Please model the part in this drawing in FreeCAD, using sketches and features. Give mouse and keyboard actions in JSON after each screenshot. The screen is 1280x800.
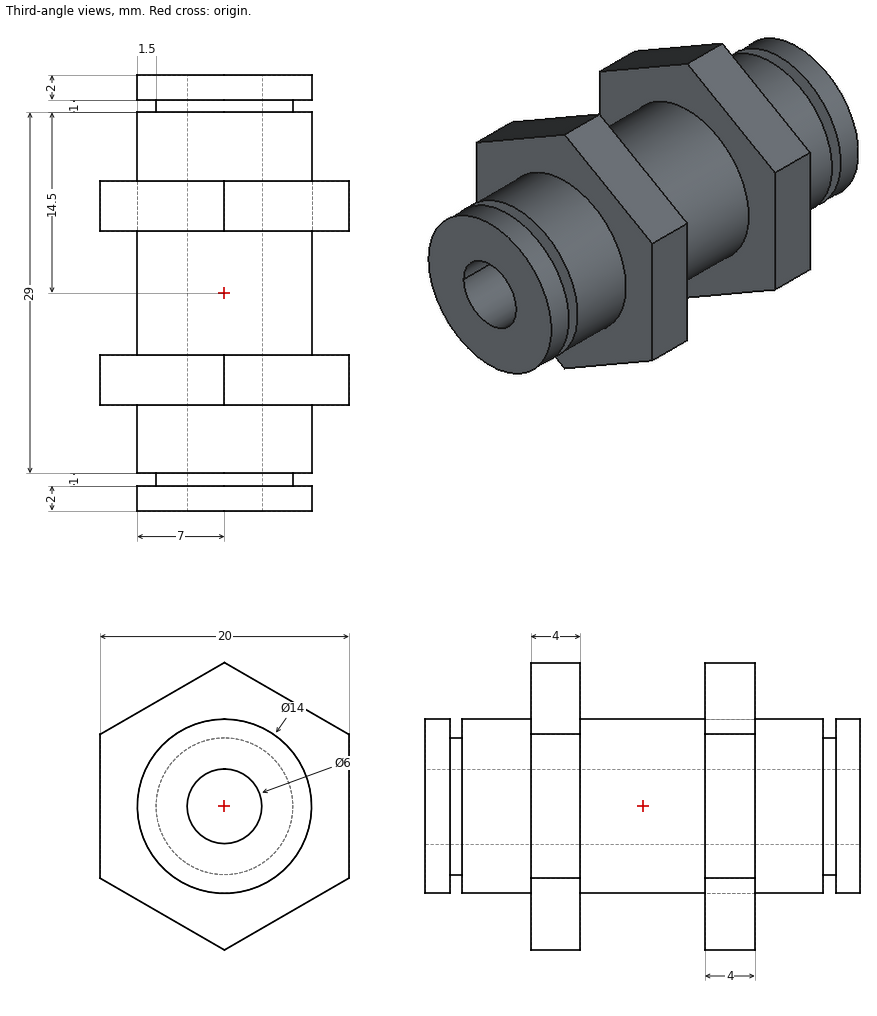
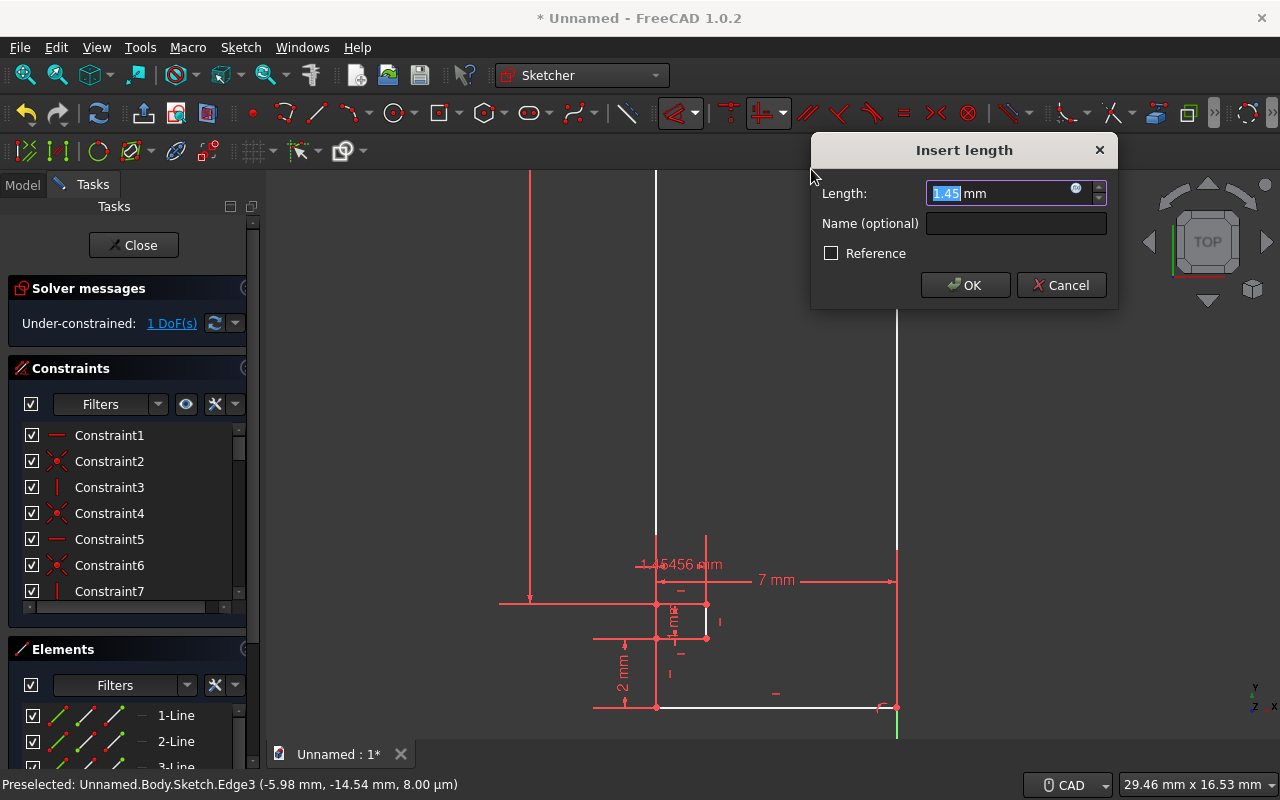
{"action": "type", "text": "1.5"}
{"action": "key", "text": "Return"}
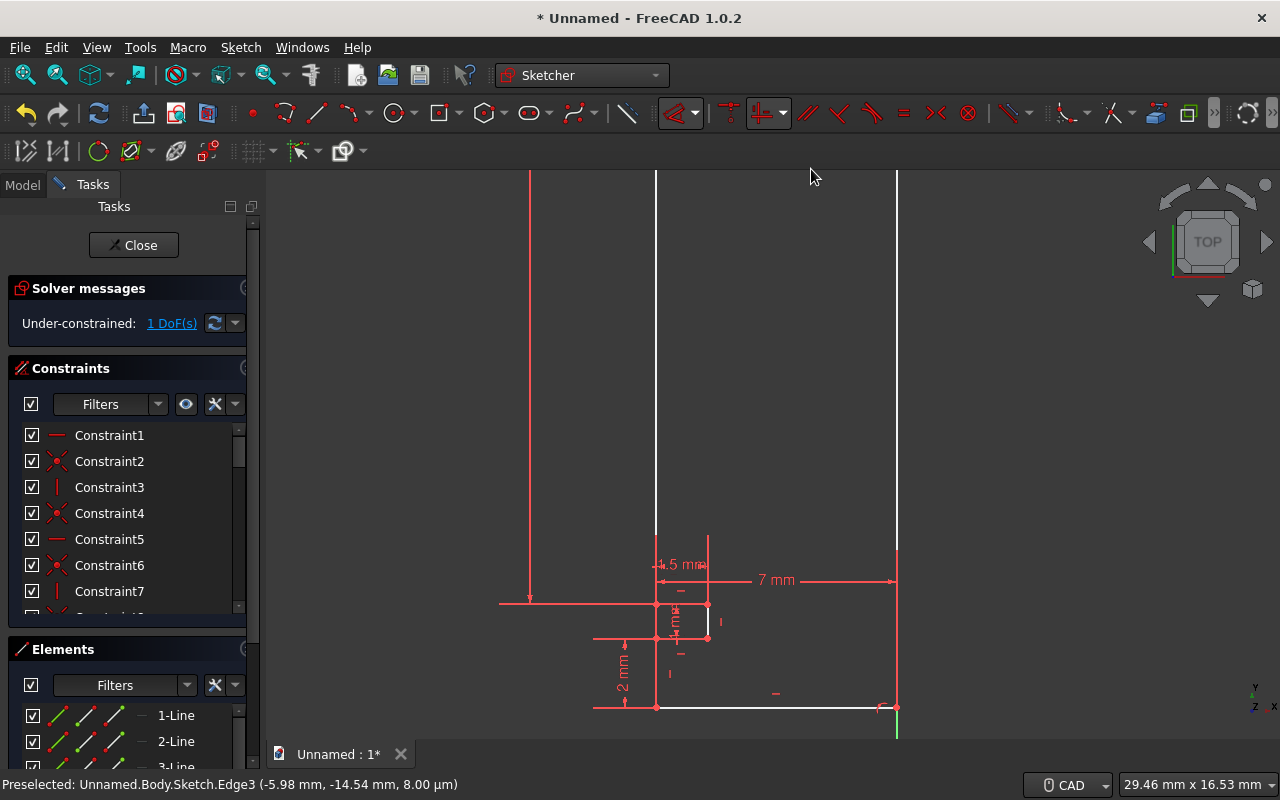
{"action": "scroll", "coordinate": [673, 606], "scroll_direction": "down", "scroll_amount": 6}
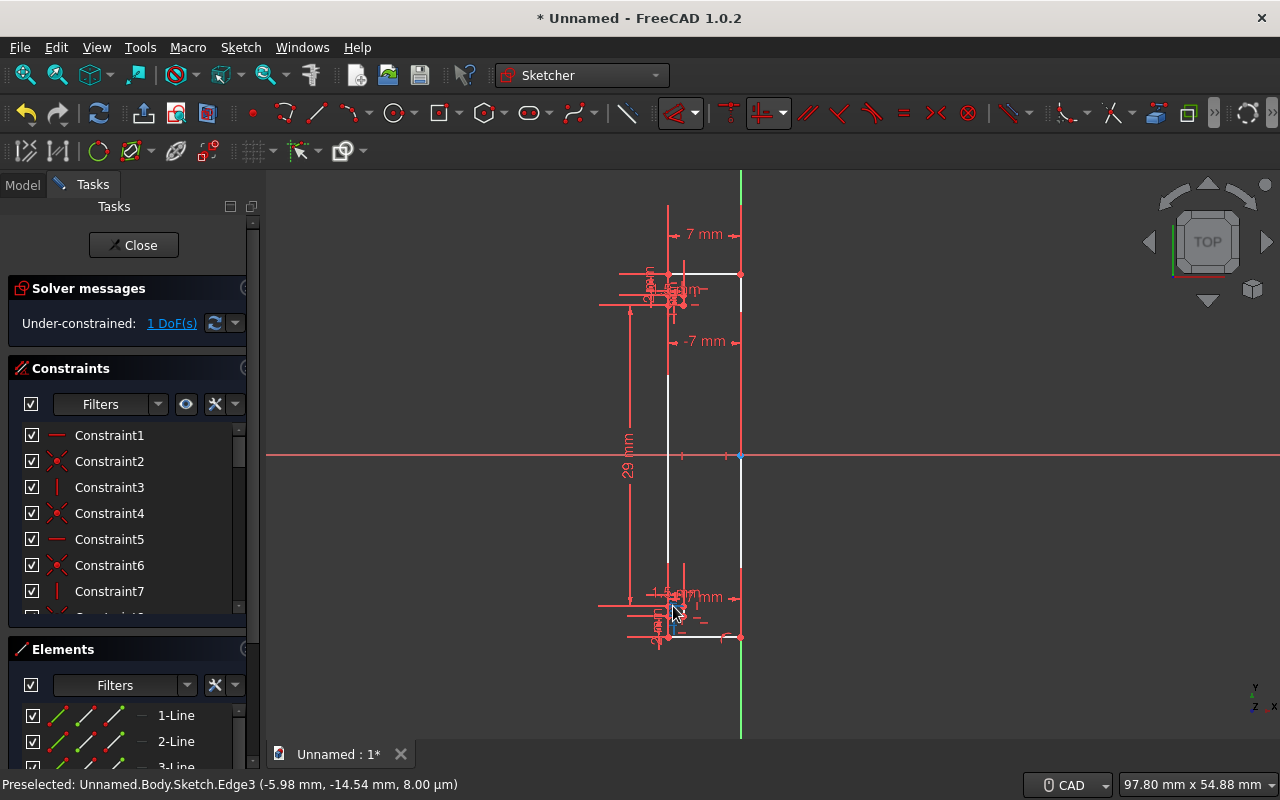
{"action": "left_click", "coordinate": [684, 305]}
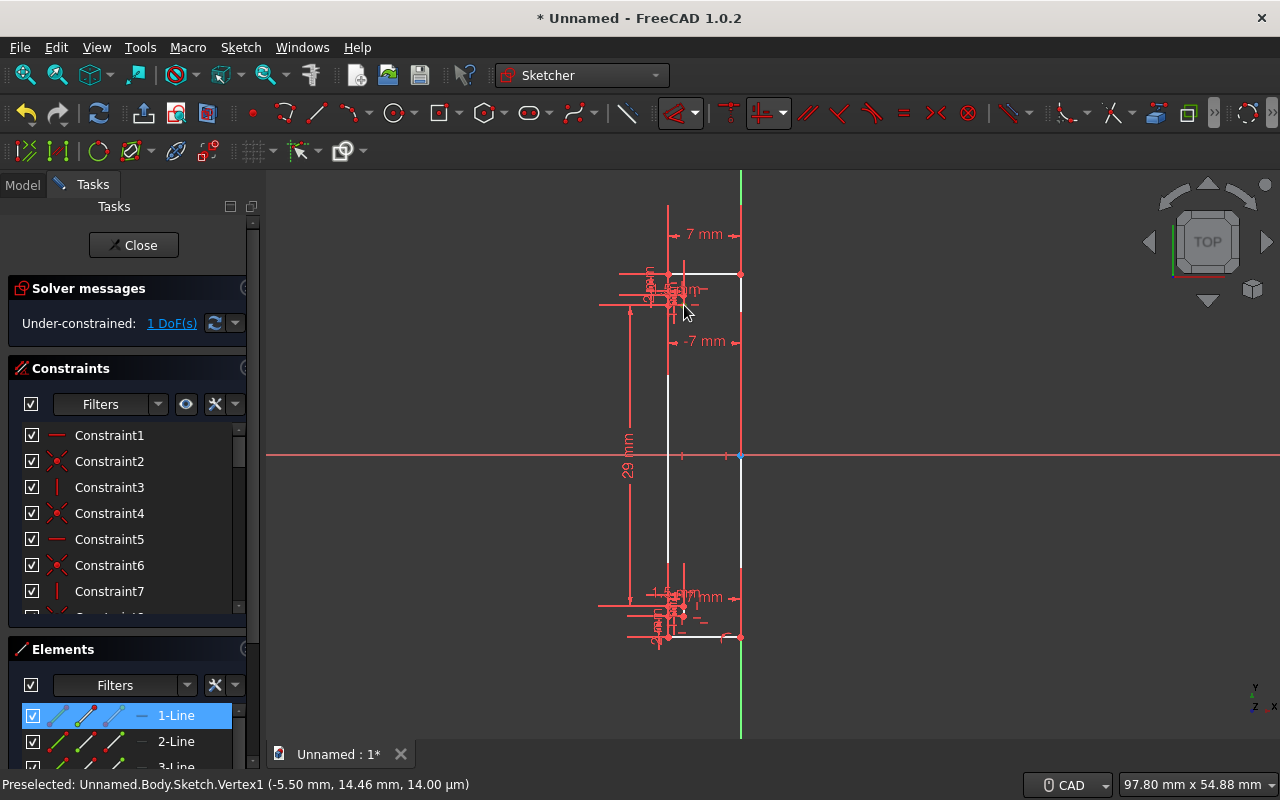
{"action": "left_click", "coordinate": [698, 114]}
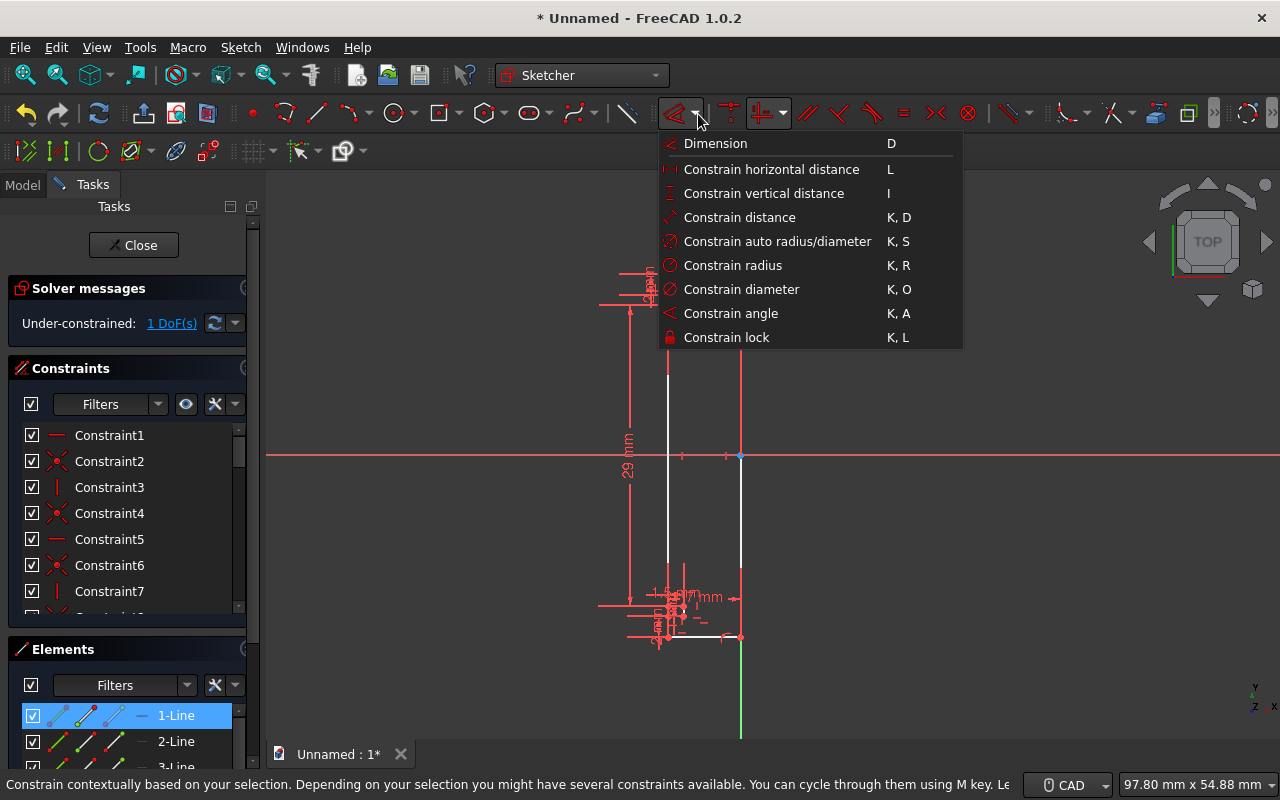
{"action": "left_click", "coordinate": [811, 193]}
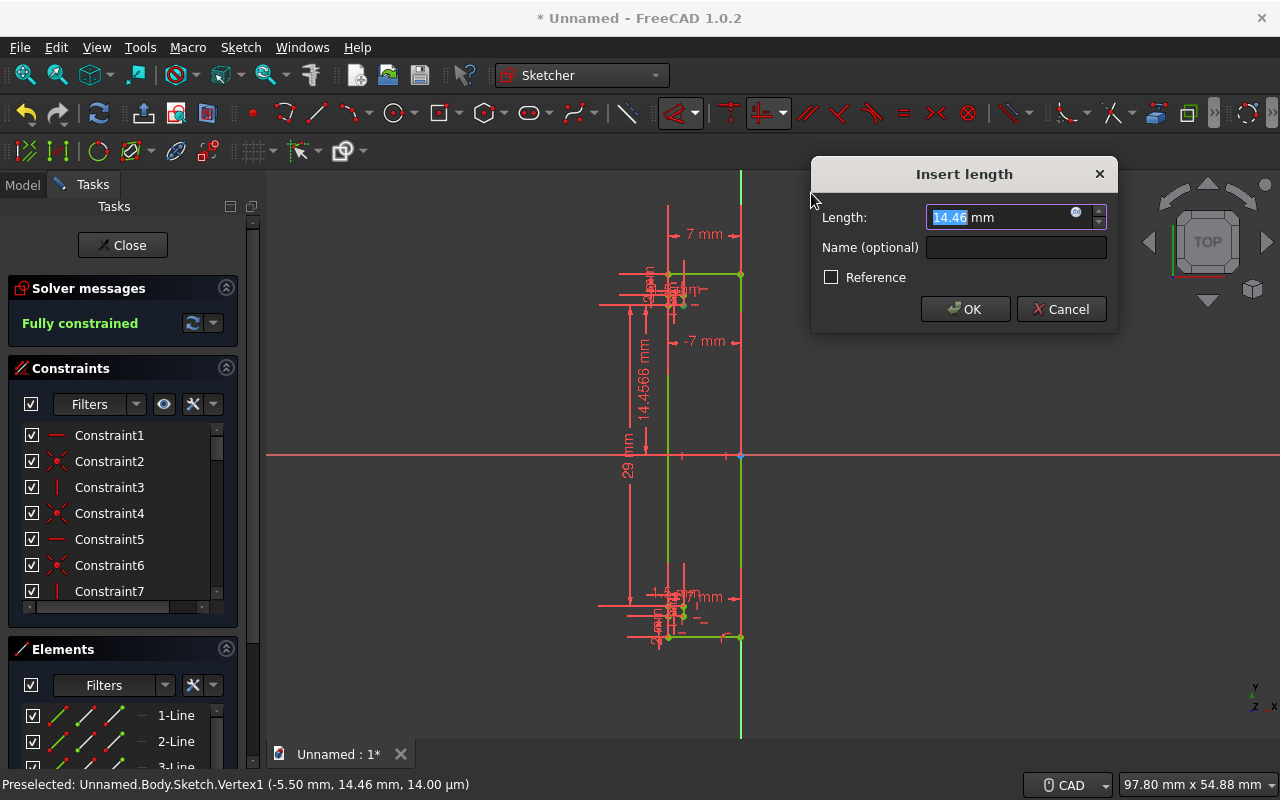
{"action": "type", "text": "14.5"}
{"action": "key", "text": "Return"}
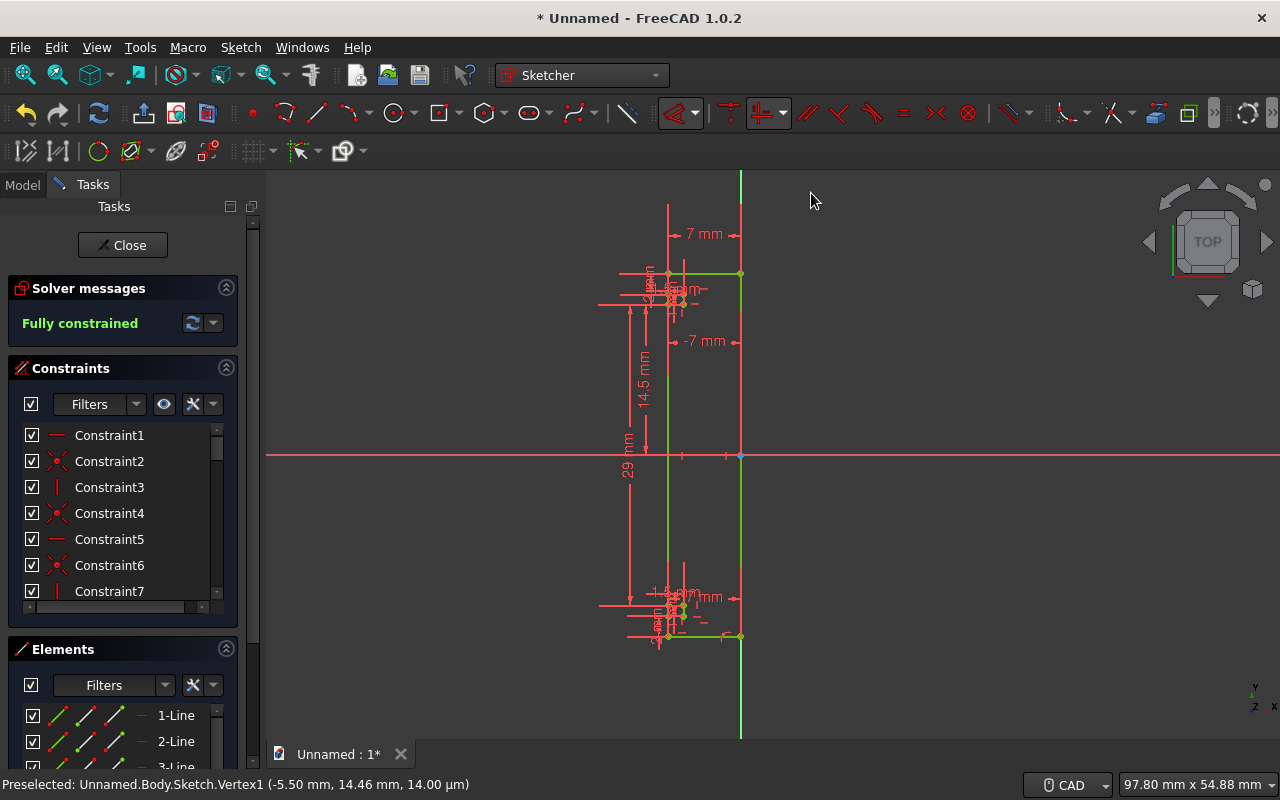
{"action": "left_click", "coordinate": [123, 245]}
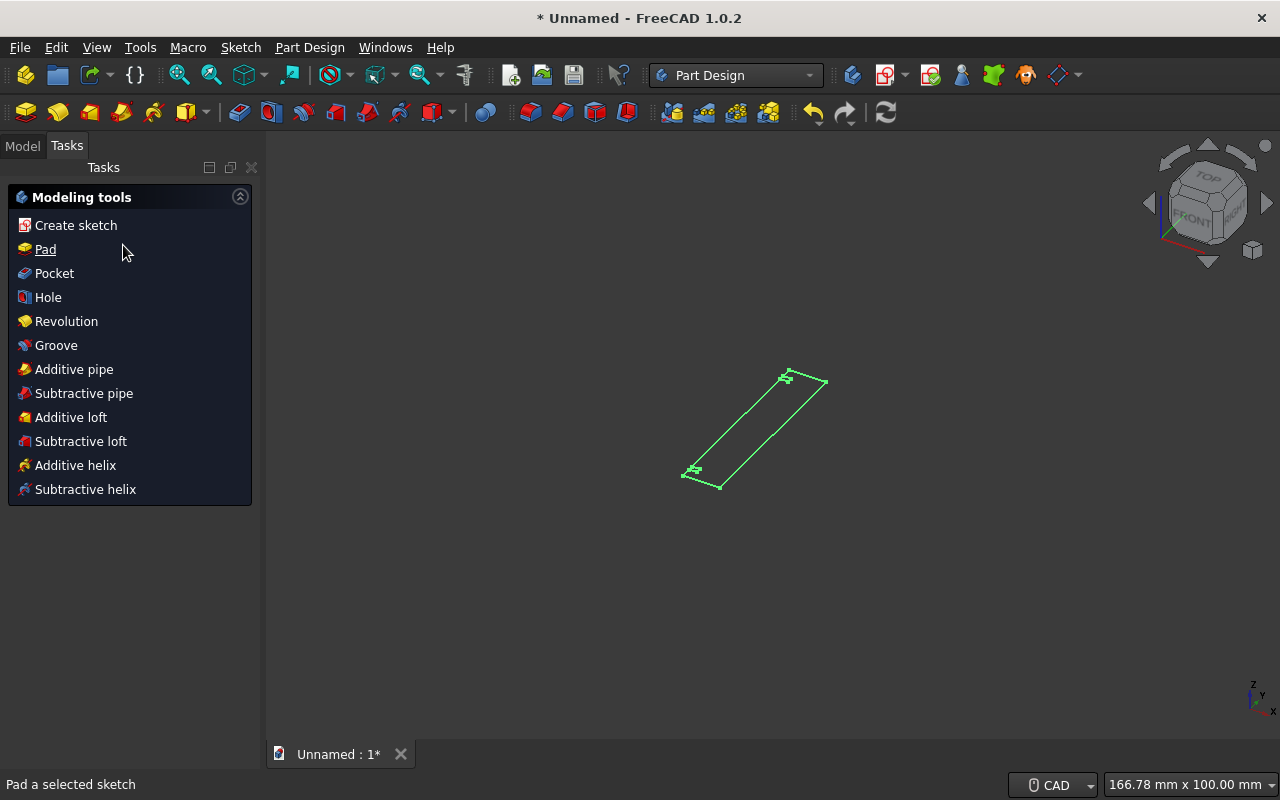
{"action": "left_click", "coordinate": [58, 112]}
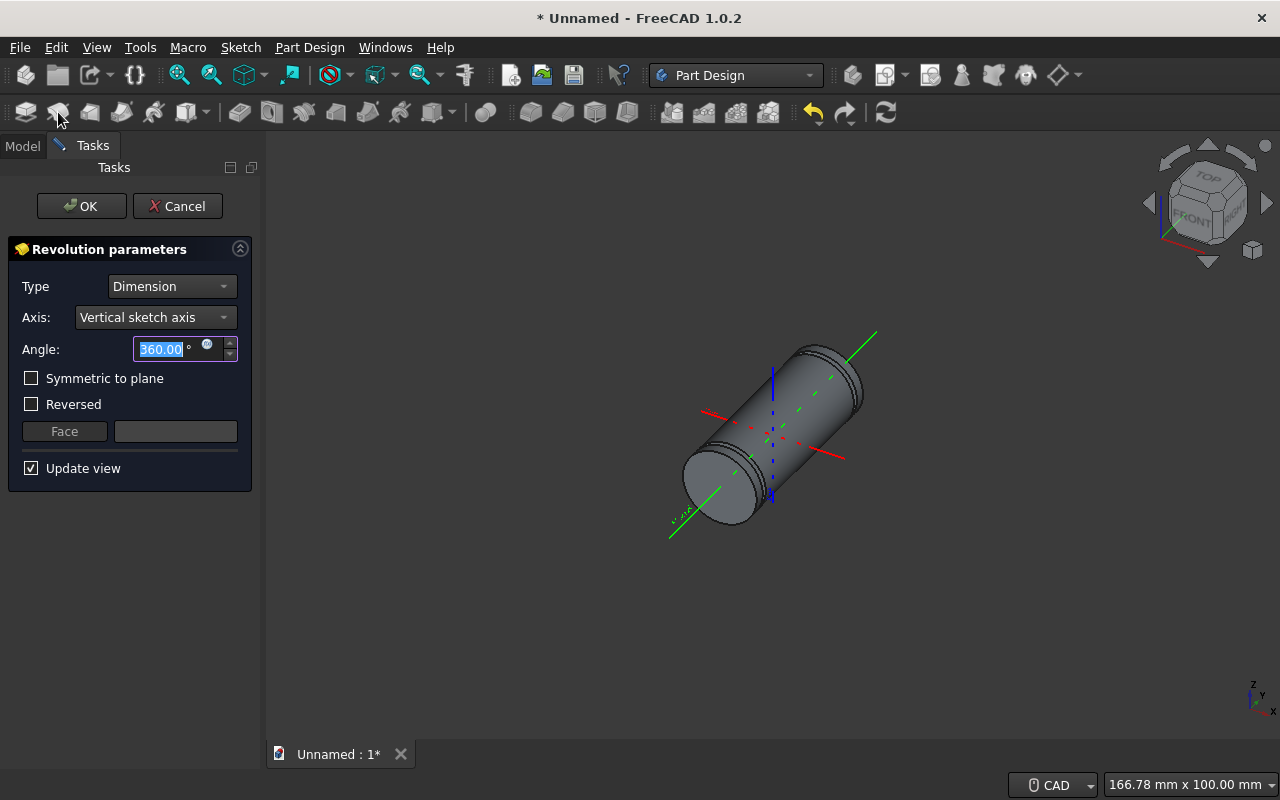
{"action": "left_click", "coordinate": [82, 206]}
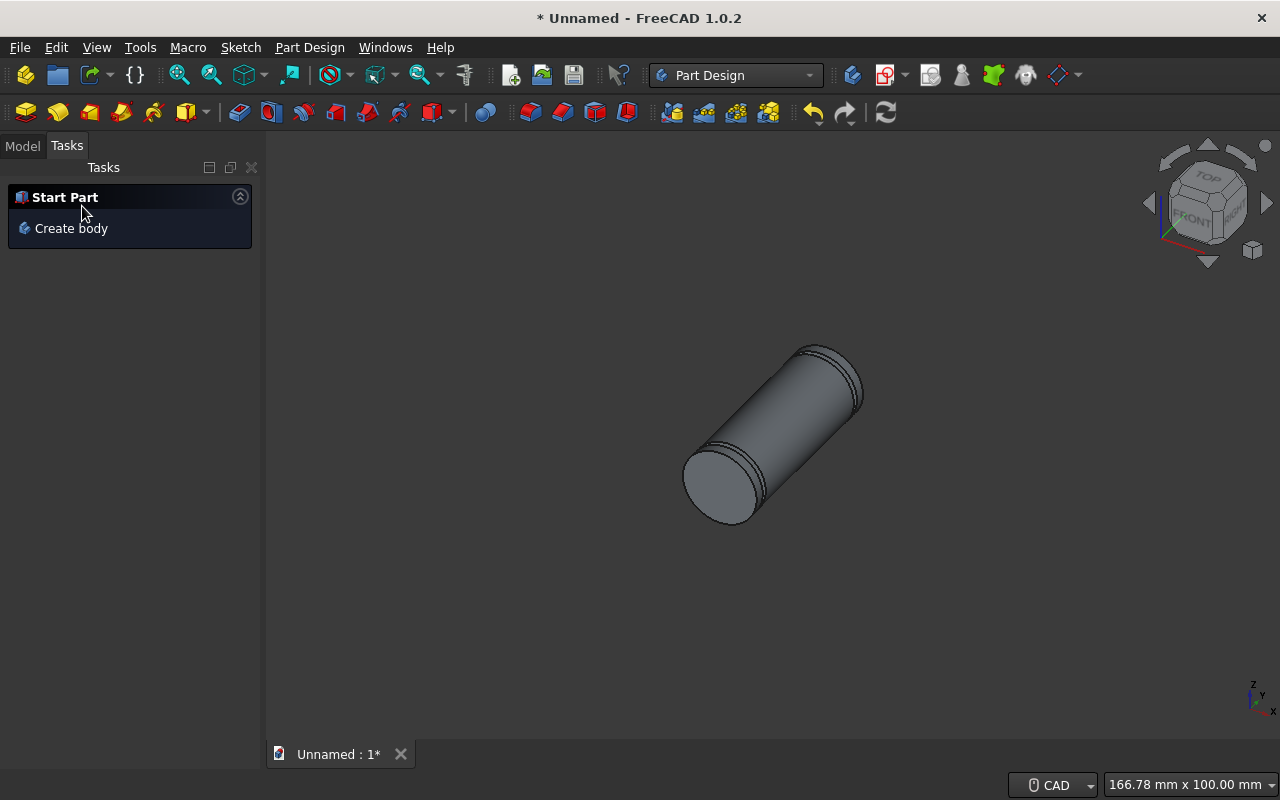
{"action": "left_click", "coordinate": [180, 76]}